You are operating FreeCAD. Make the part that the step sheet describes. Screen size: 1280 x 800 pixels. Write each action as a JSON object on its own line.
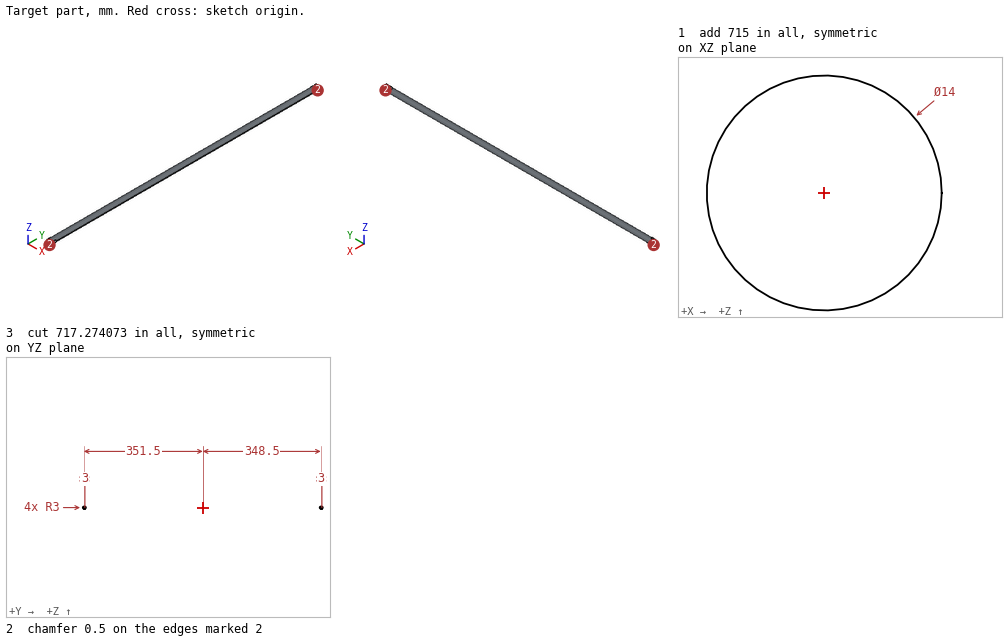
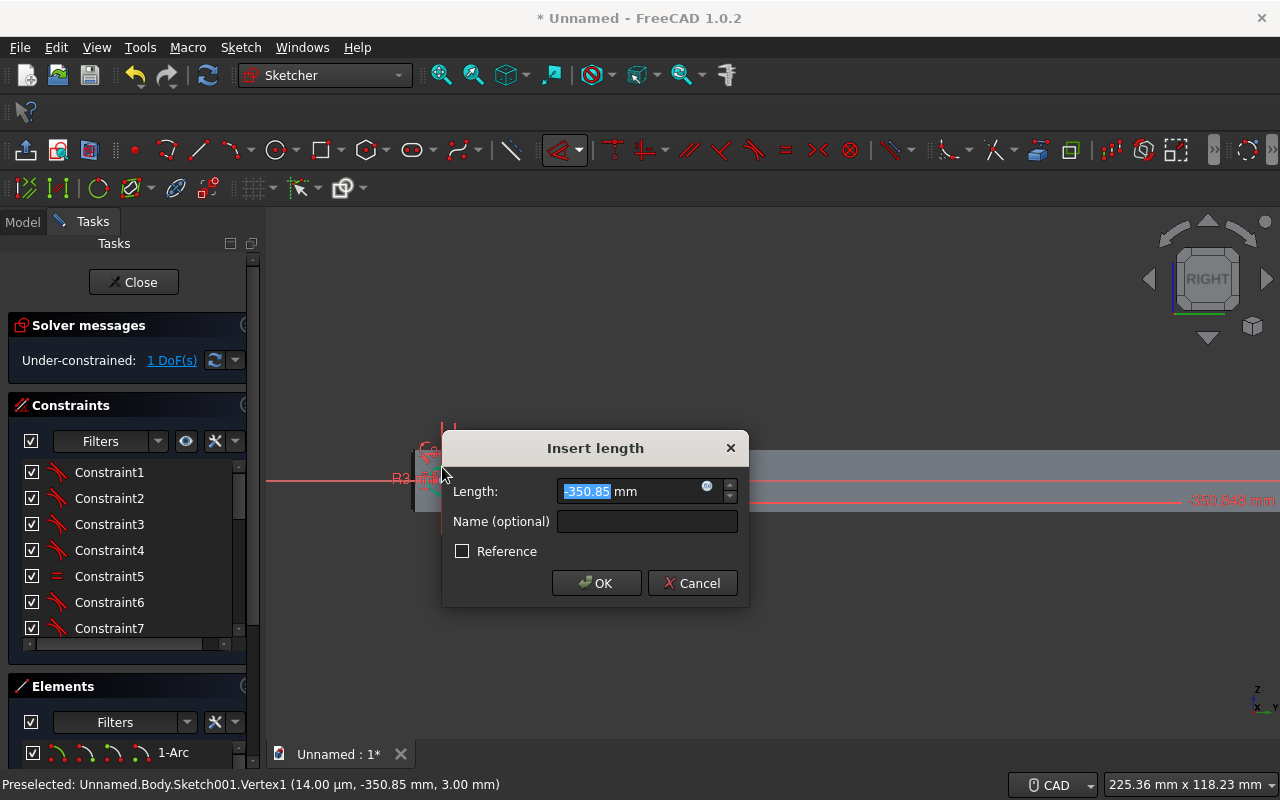
{"action": "type", "text": "-351.5"}
{"action": "key", "text": "Return"}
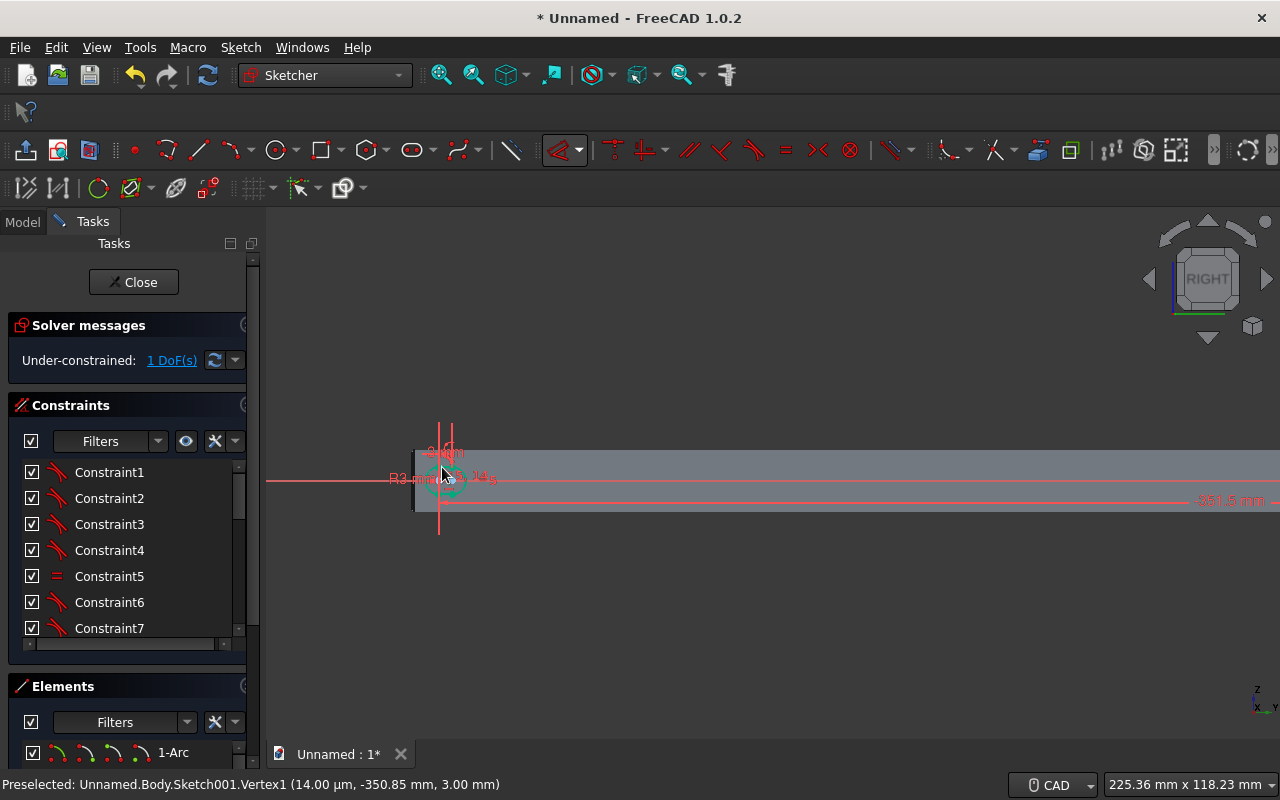
{"action": "scroll", "coordinate": [444, 471], "scroll_direction": "down", "scroll_amount": 9}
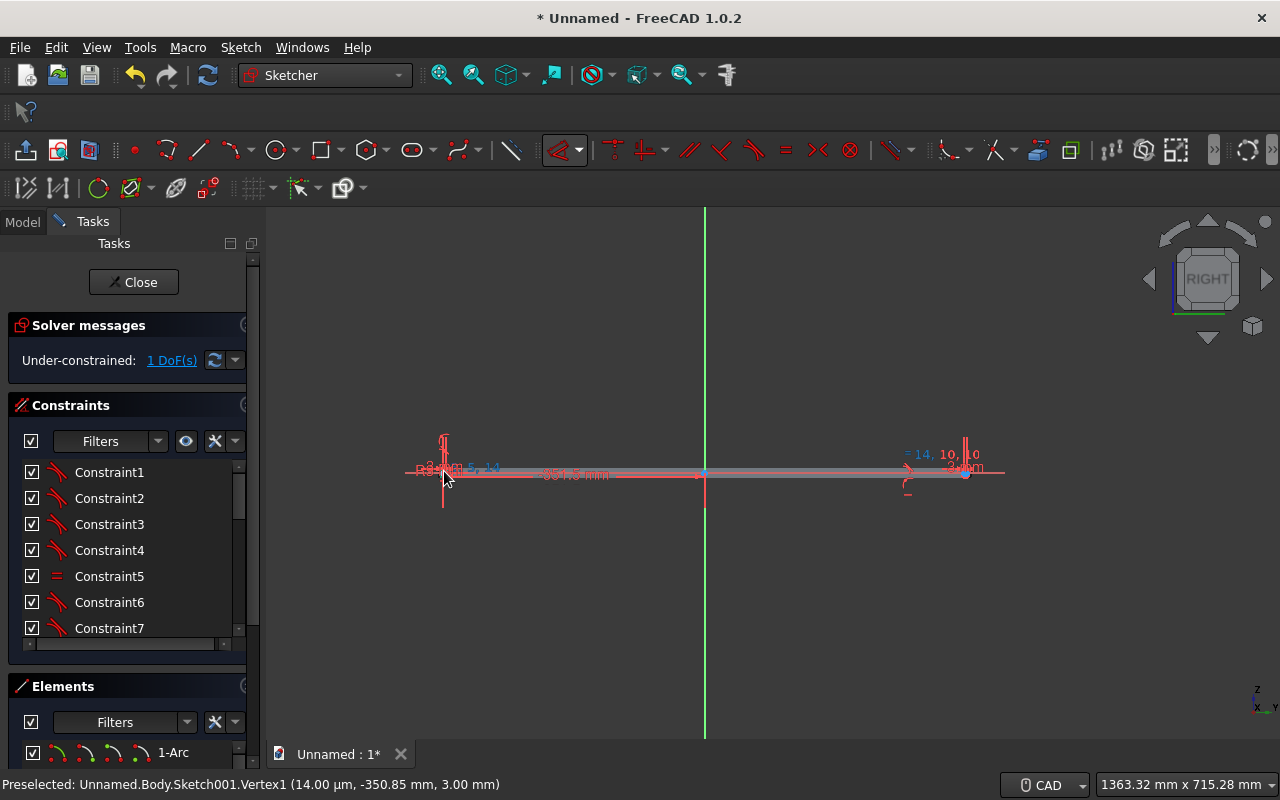
{"action": "scroll", "coordinate": [964, 471], "scroll_direction": "up", "scroll_amount": 9}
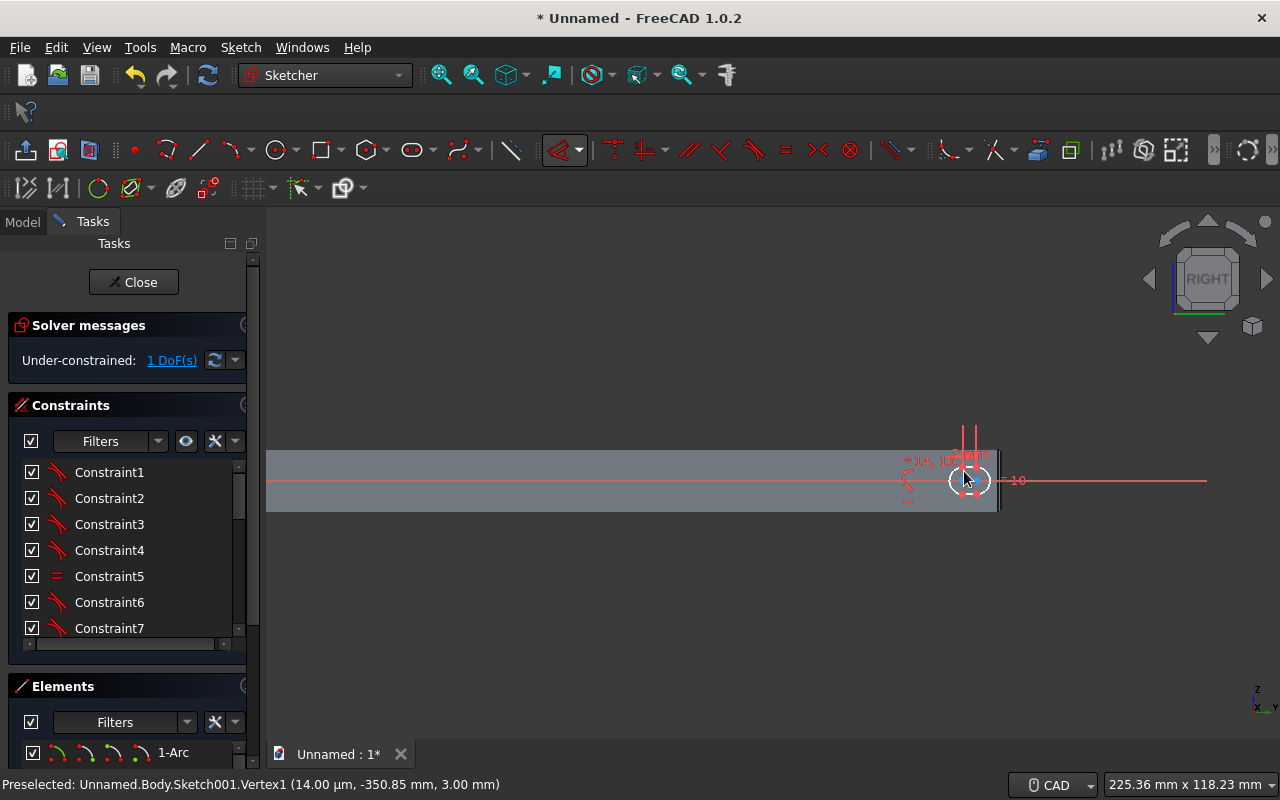
{"action": "left_click", "coordinate": [963, 467]}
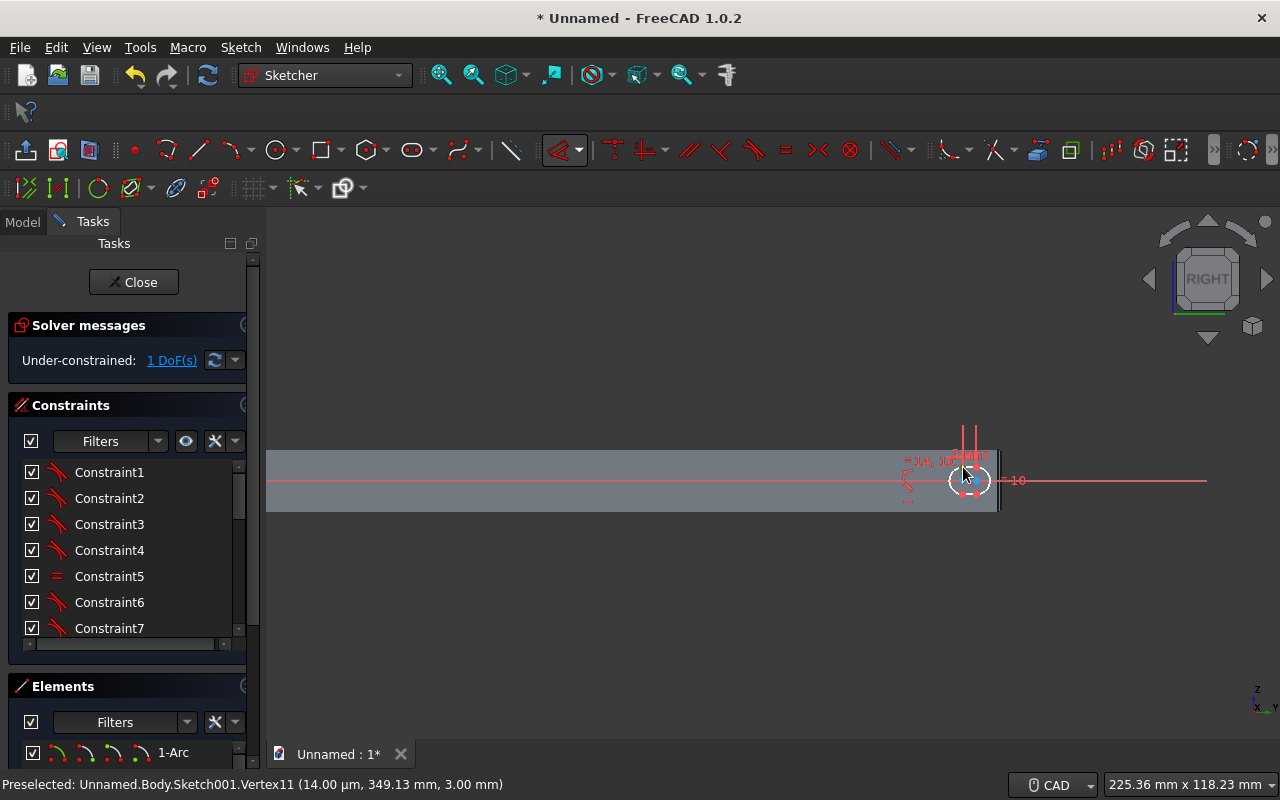
{"action": "key", "text": "l"}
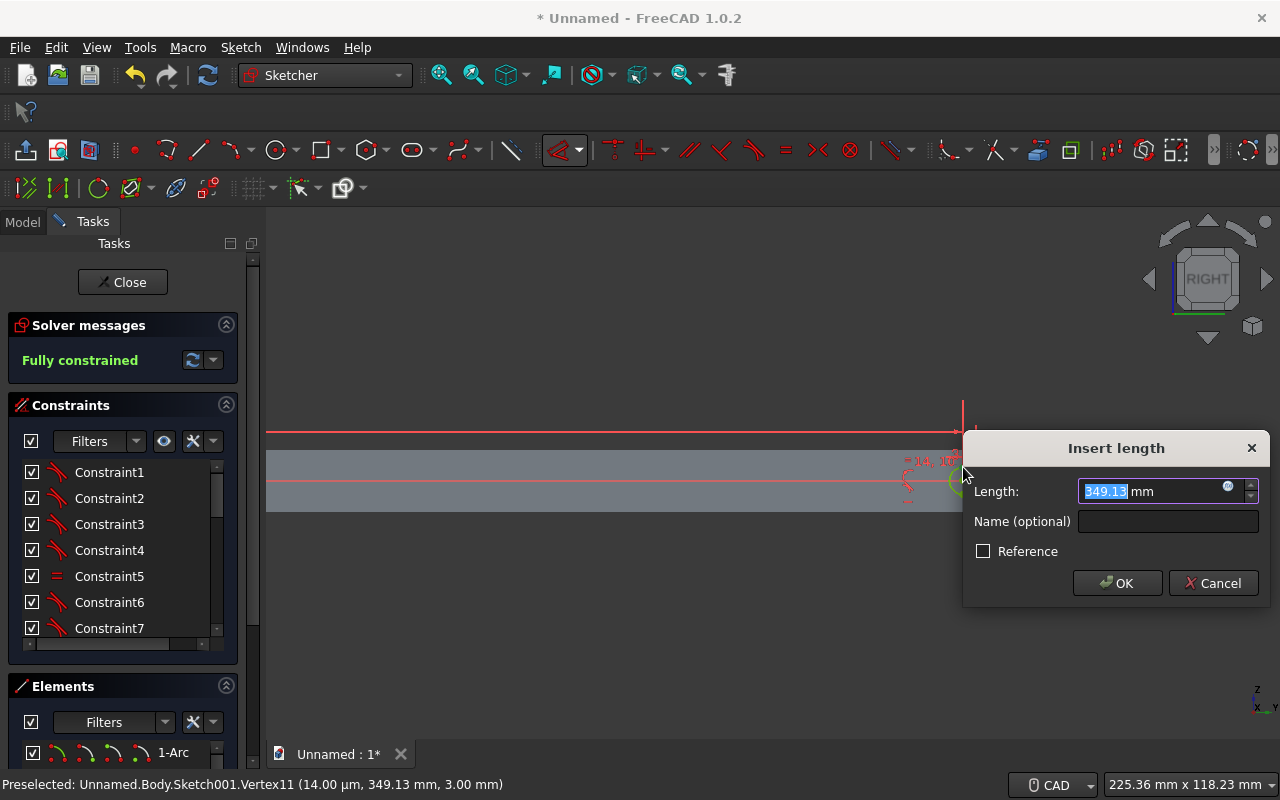
{"action": "type", "text": "348.5"}
{"action": "key", "text": "Return"}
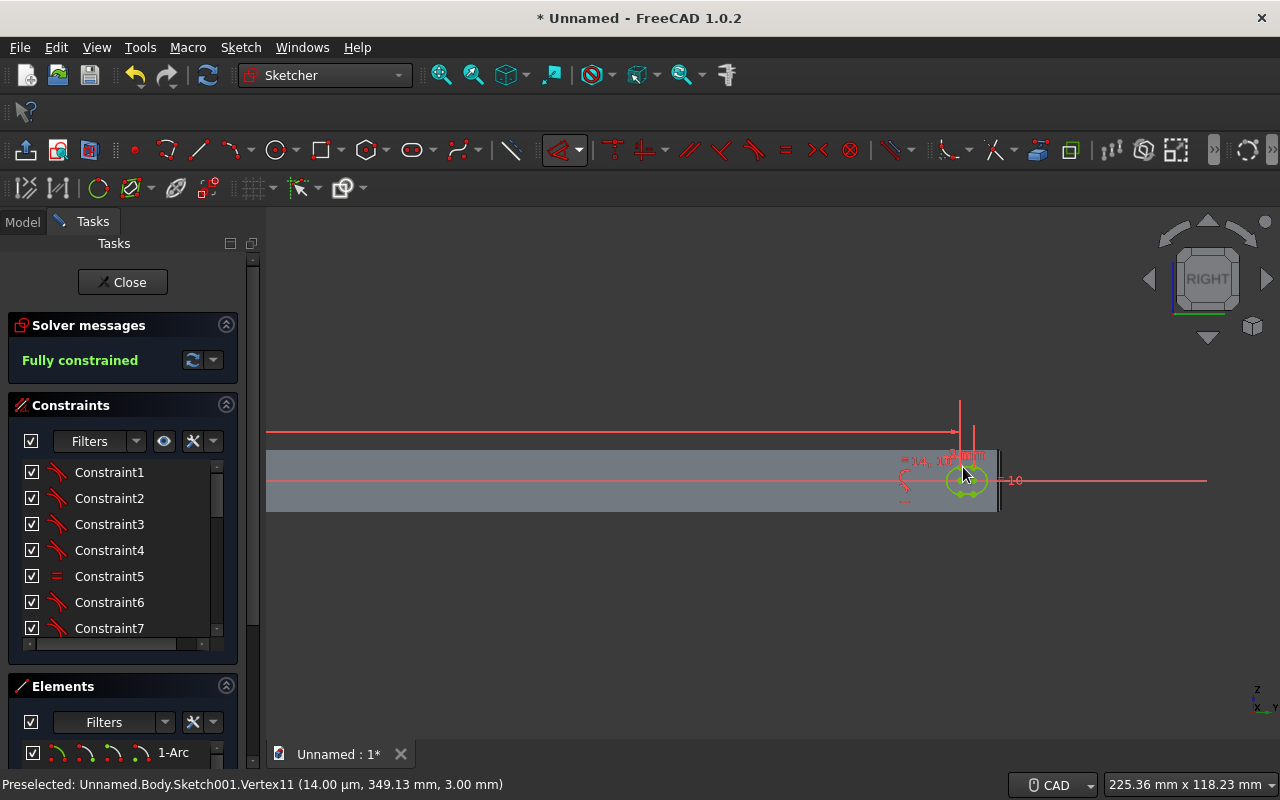
{"action": "left_click", "coordinate": [123, 282]}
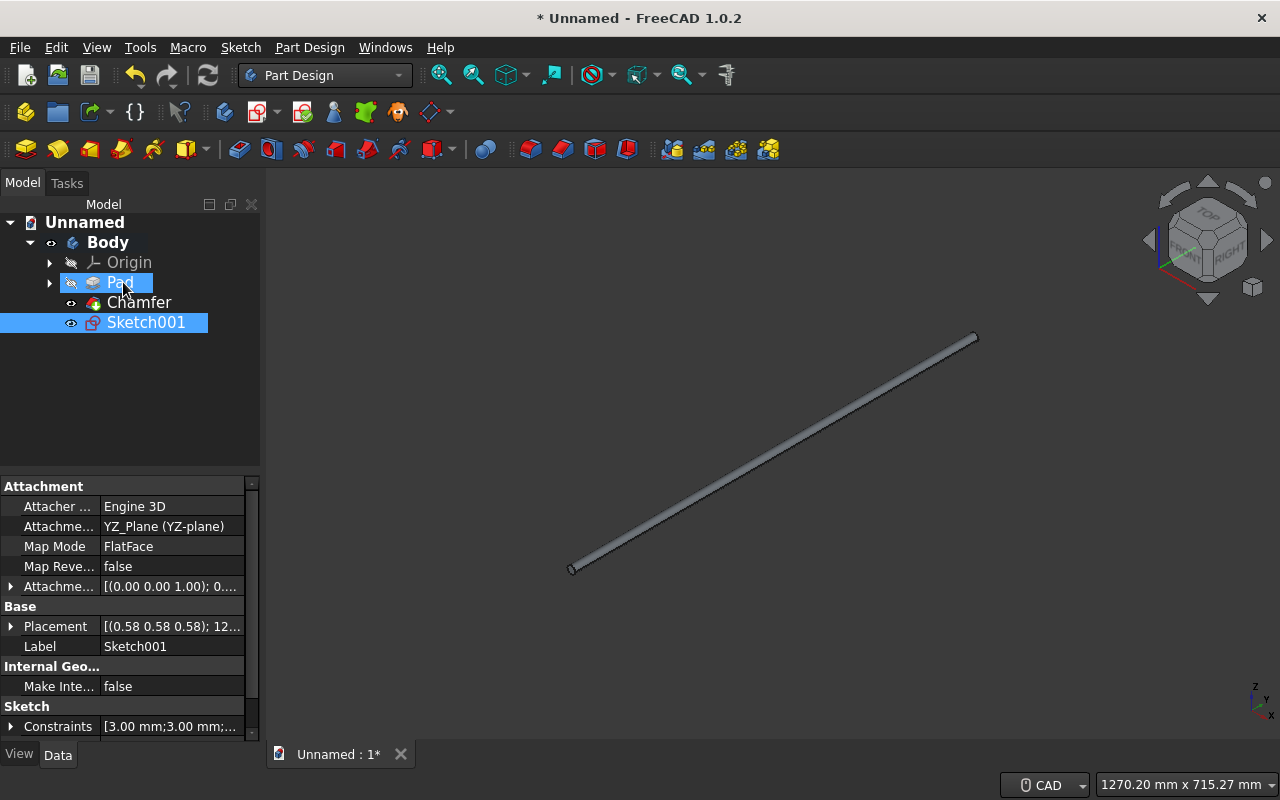
{"action": "left_click", "coordinate": [240, 150]}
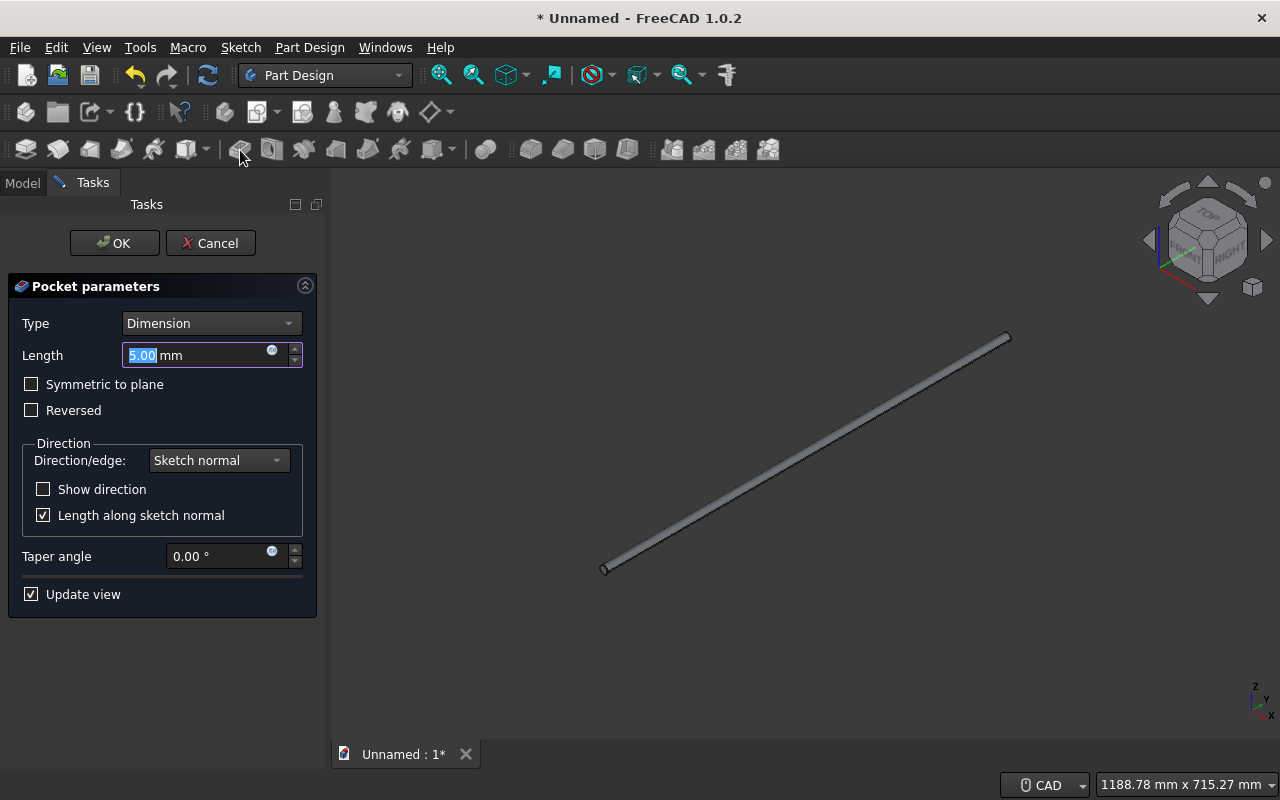
{"action": "type", "text": "717.274073"}
{"action": "key", "text": "Tab"}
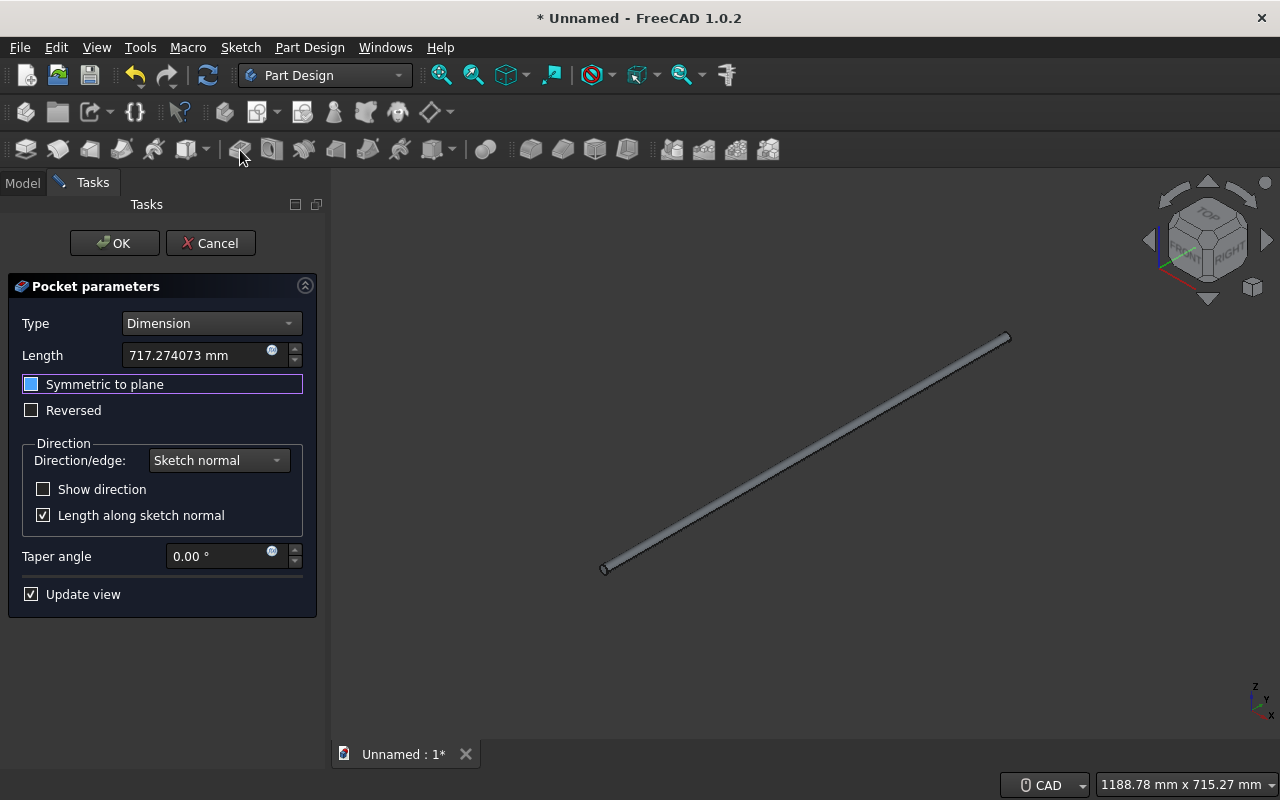
{"action": "left_click", "coordinate": [30, 384]}